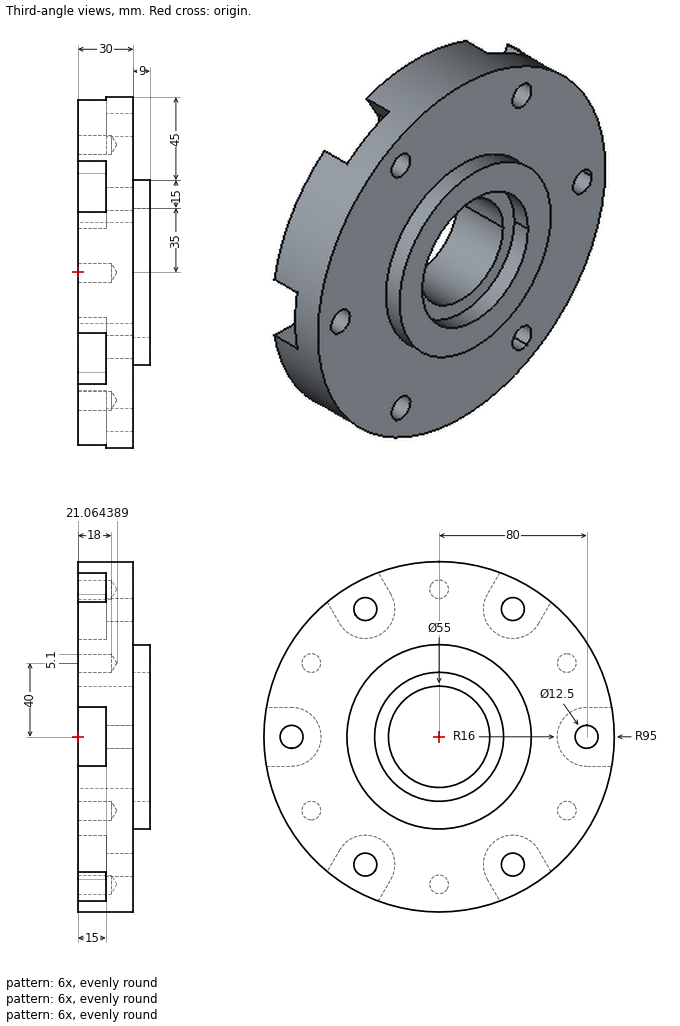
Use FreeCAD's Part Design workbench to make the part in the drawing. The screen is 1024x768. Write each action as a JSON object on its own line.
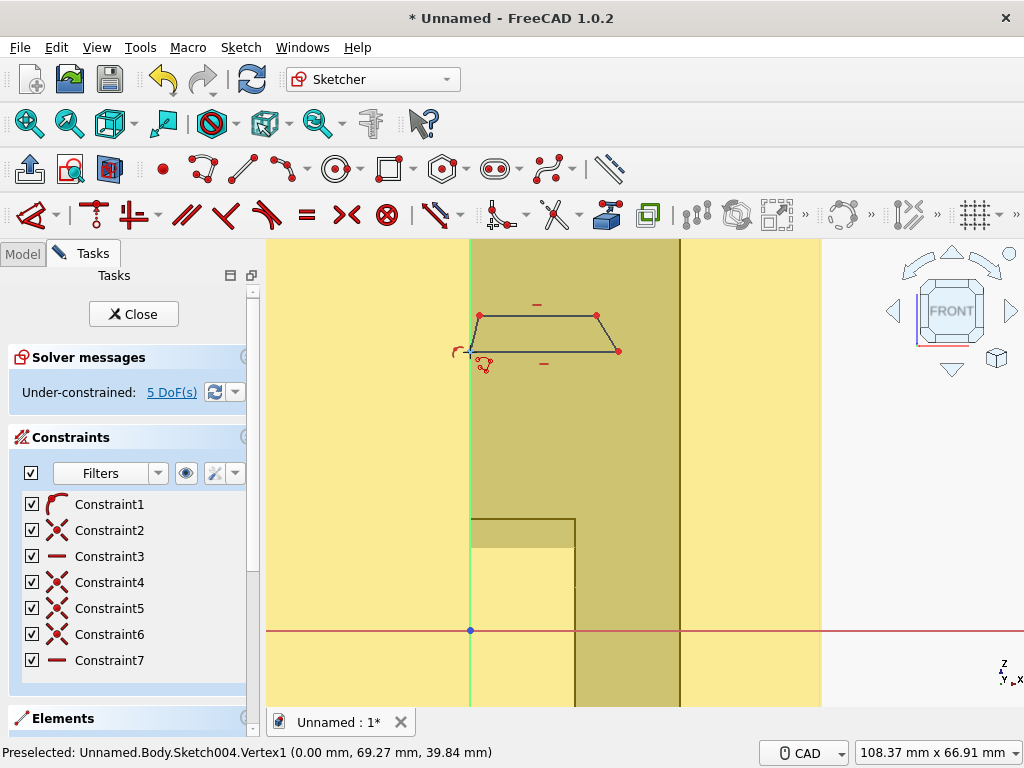
{"action": "left_click", "coordinate": [244, 170]}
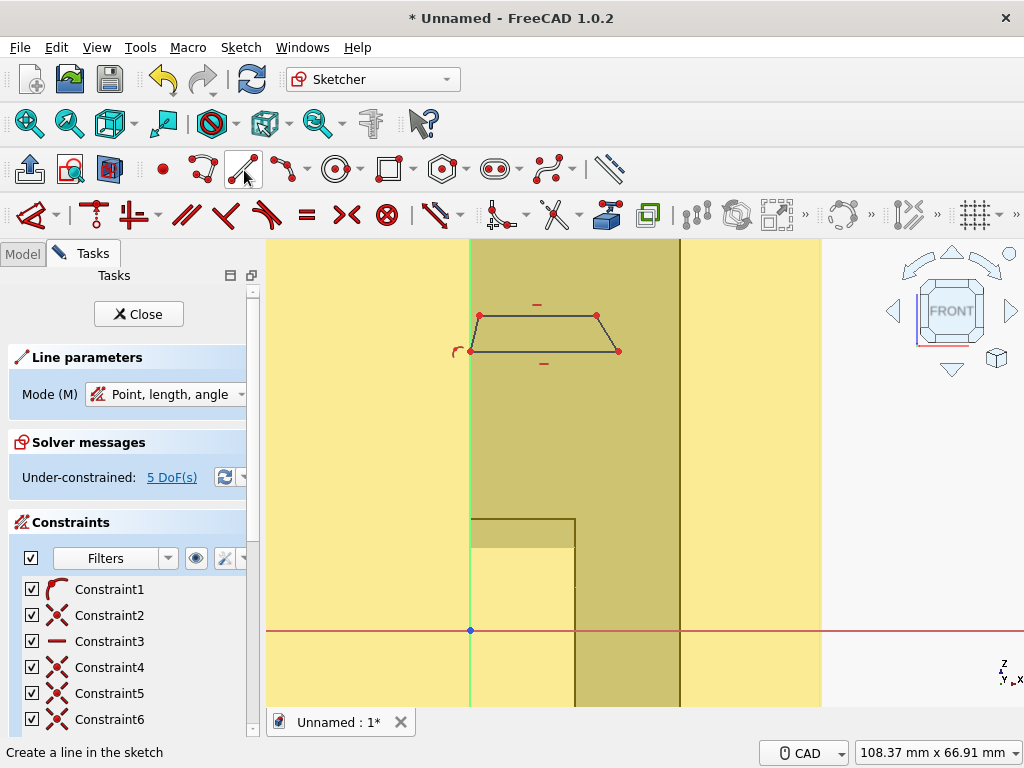
{"action": "left_click", "coordinate": [632, 351]}
{"action": "left_click", "coordinate": [677, 351]}
{"action": "key", "text": "Escape"}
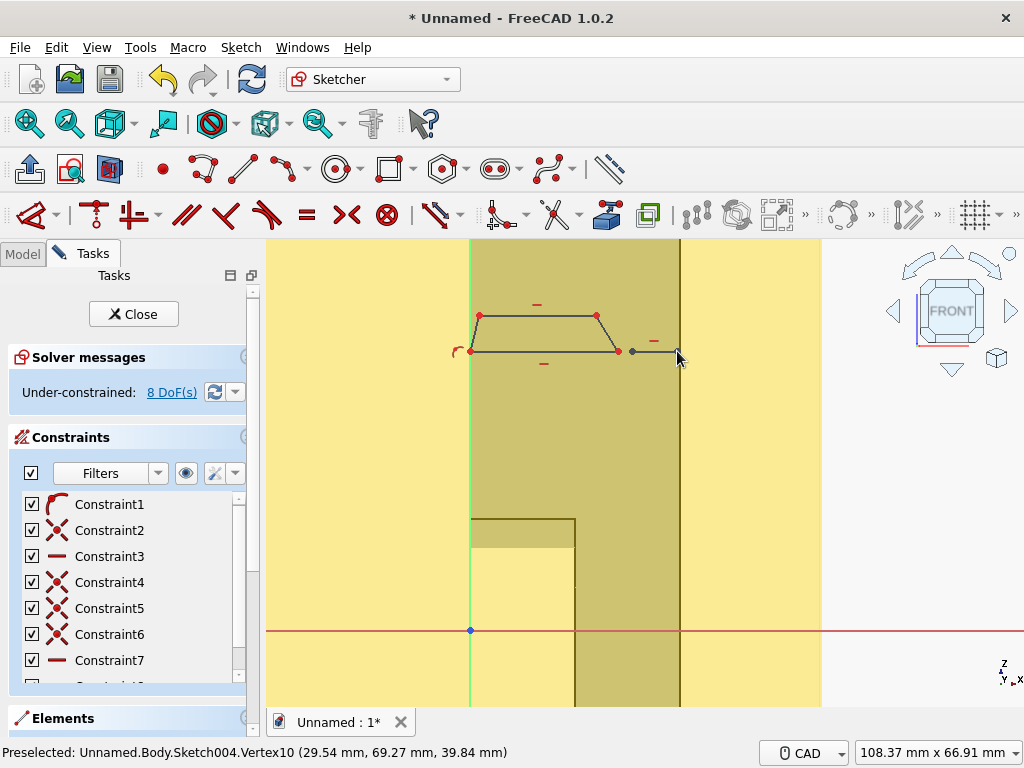
{"action": "left_click", "coordinate": [645, 352]}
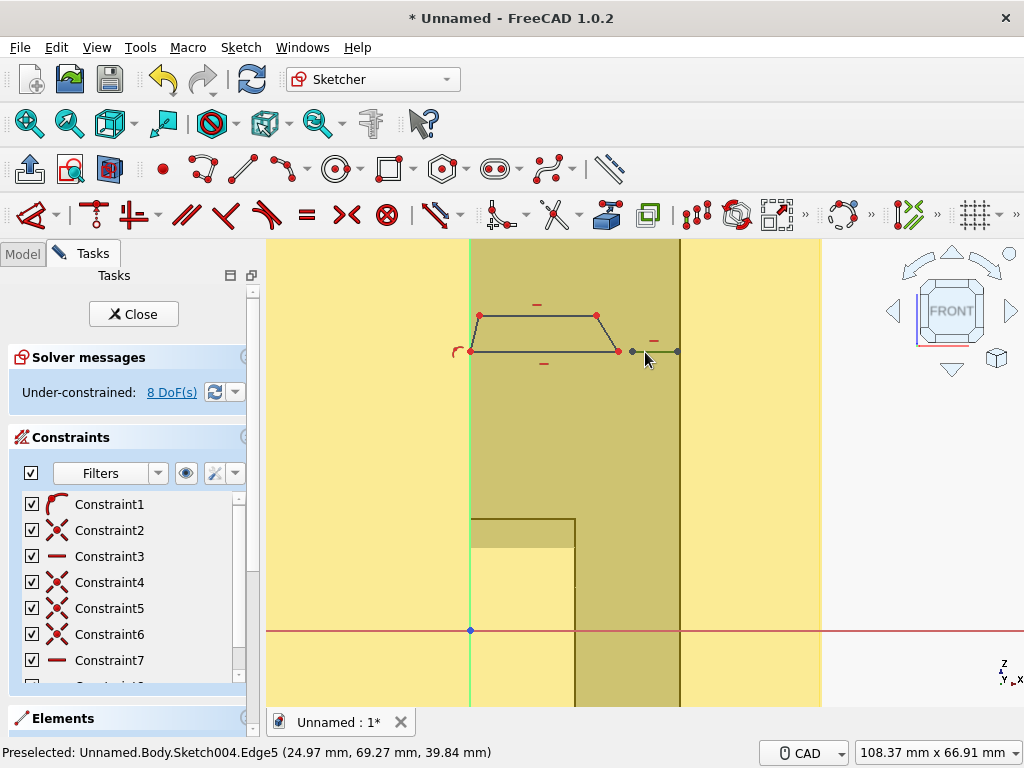
{"action": "left_click", "coordinate": [610, 170]}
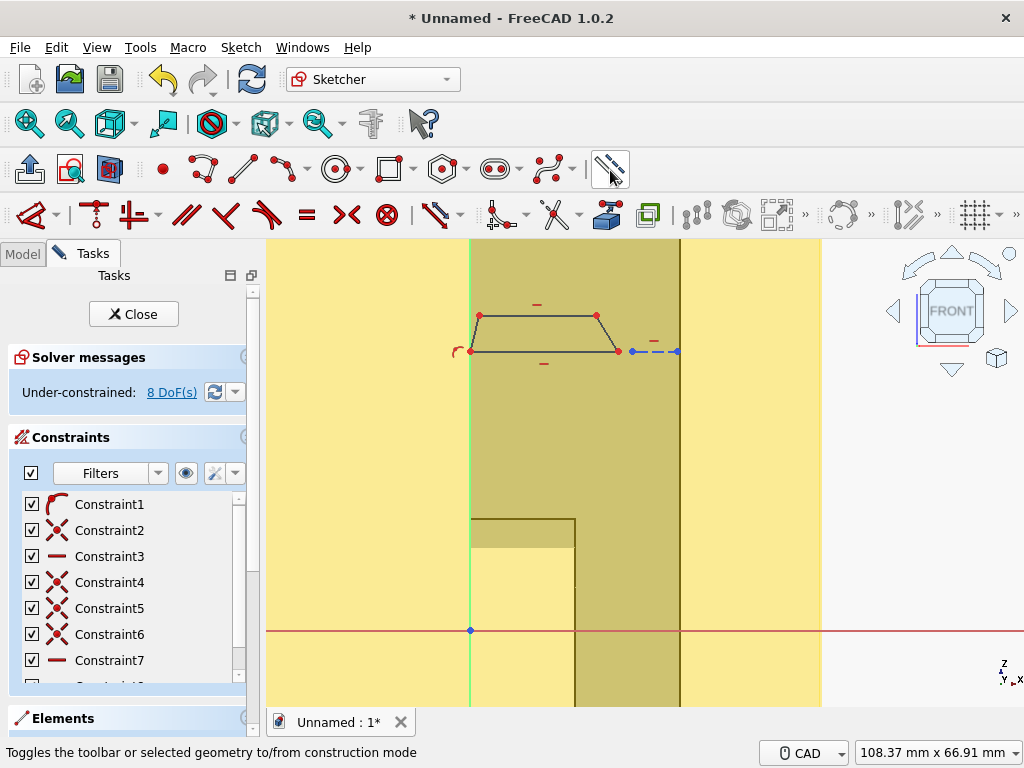
{"action": "scroll", "coordinate": [473, 341], "scroll_direction": "up", "scroll_amount": 2}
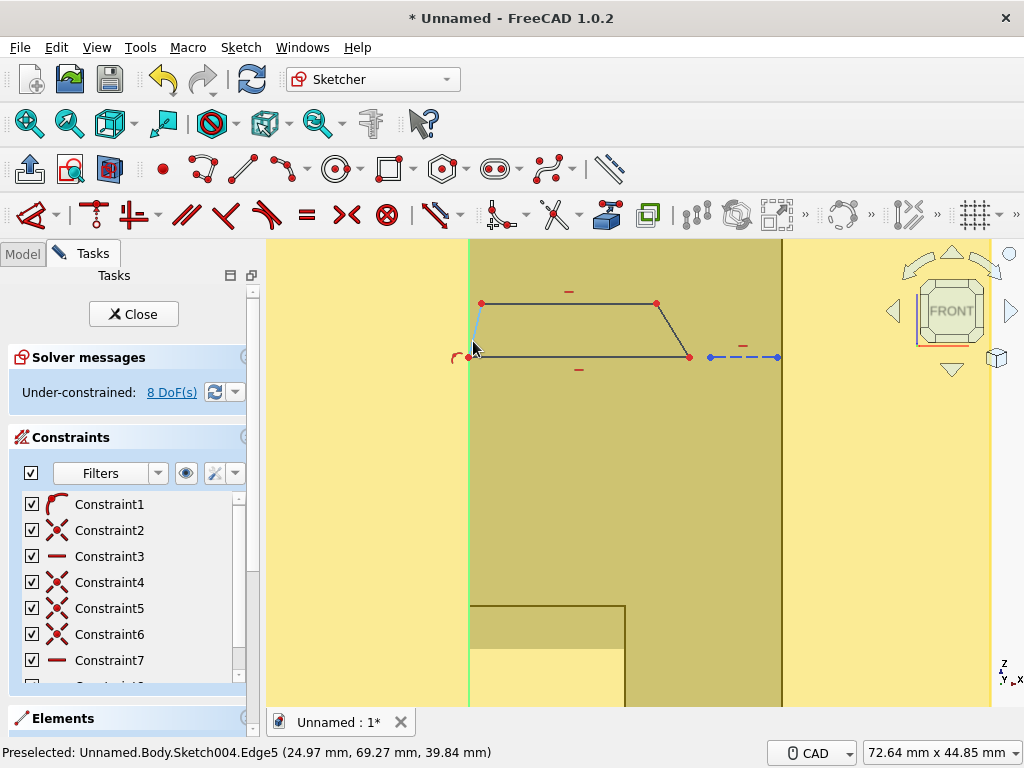
{"action": "left_click", "coordinate": [473, 341]}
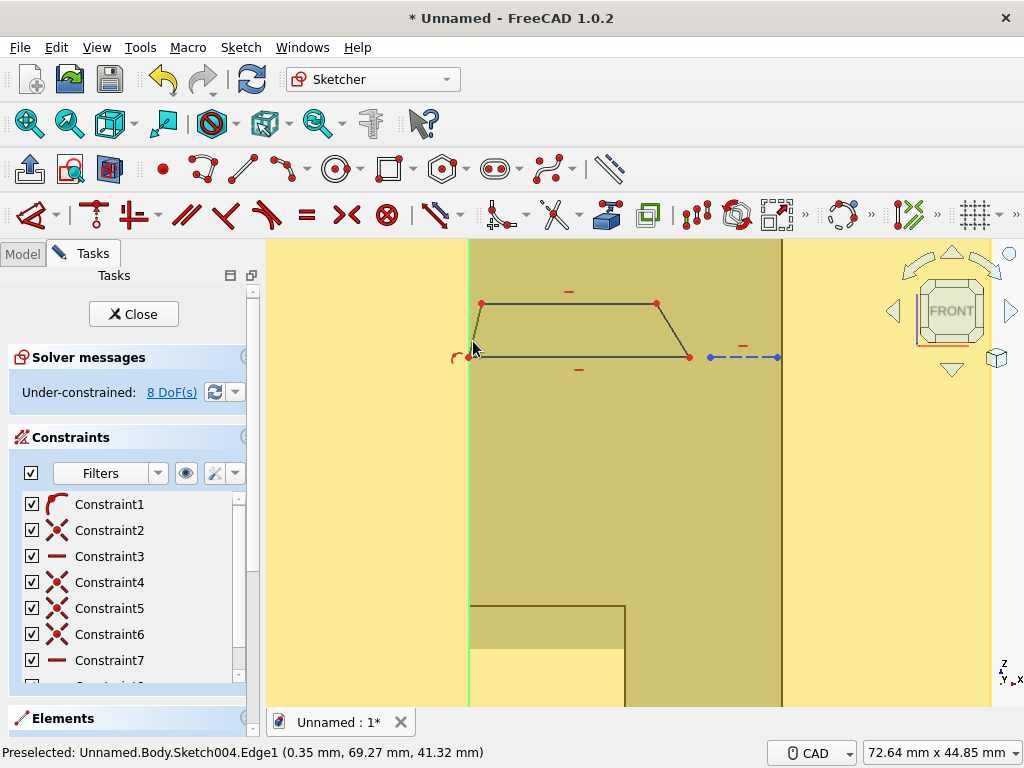
{"action": "left_click", "coordinate": [160, 216]}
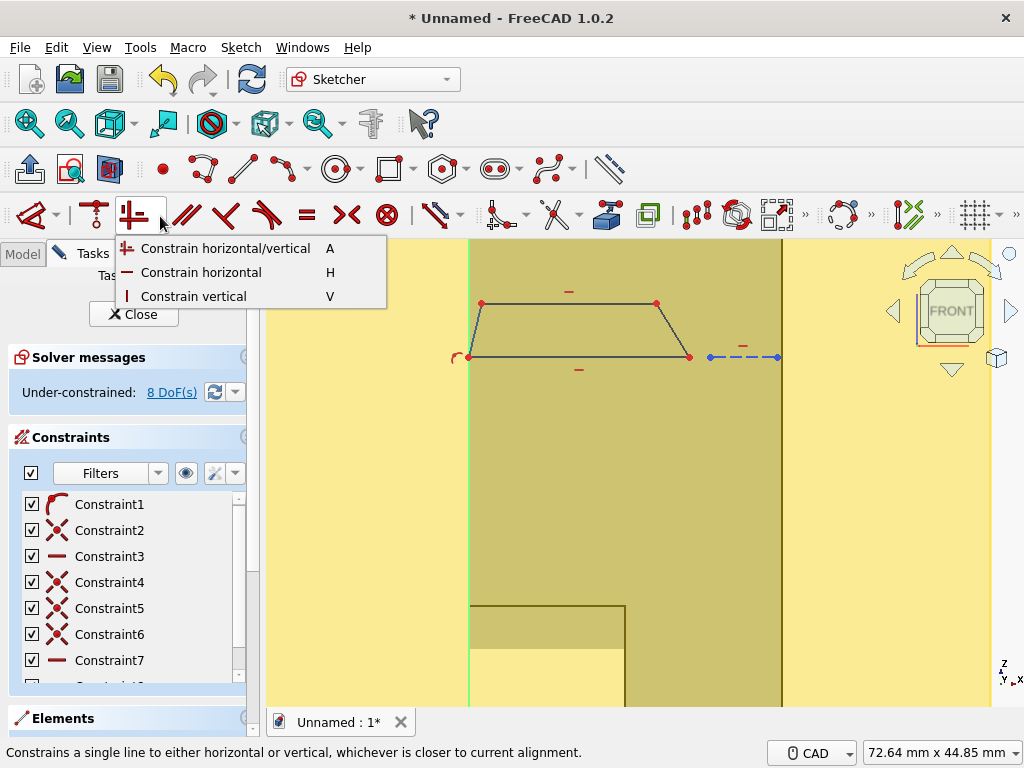
{"action": "left_click", "coordinate": [251, 296]}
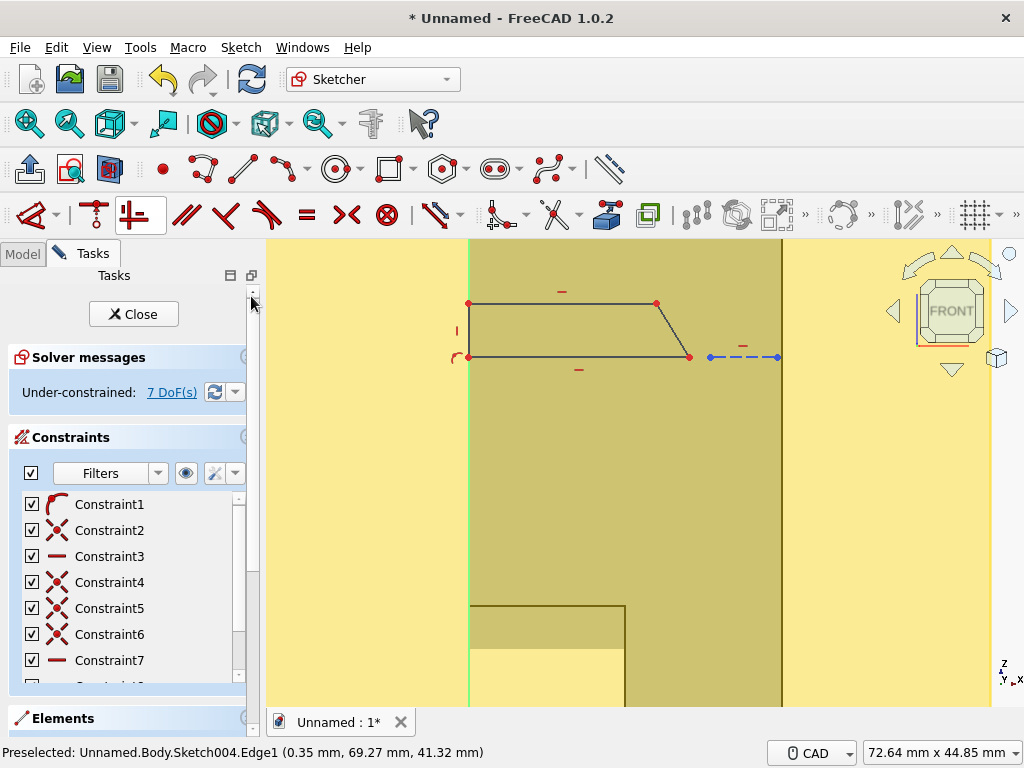
{"action": "key", "text": "d"}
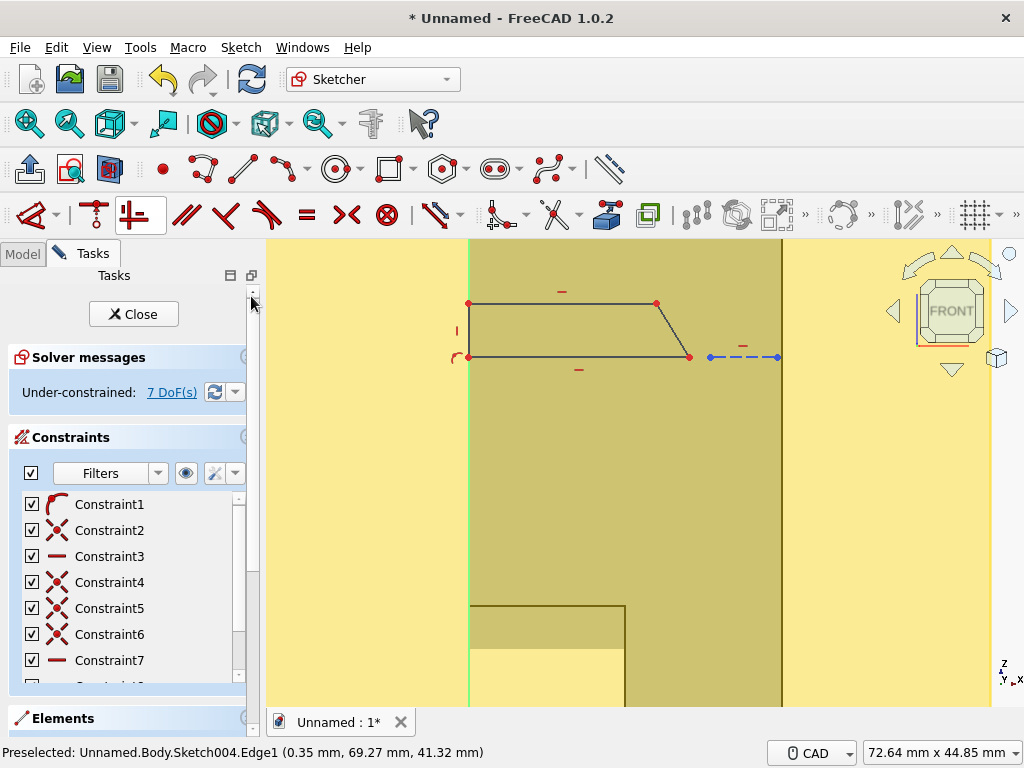
{"action": "left_click", "coordinate": [525, 304]}
{"action": "left_click", "coordinate": [563, 270]}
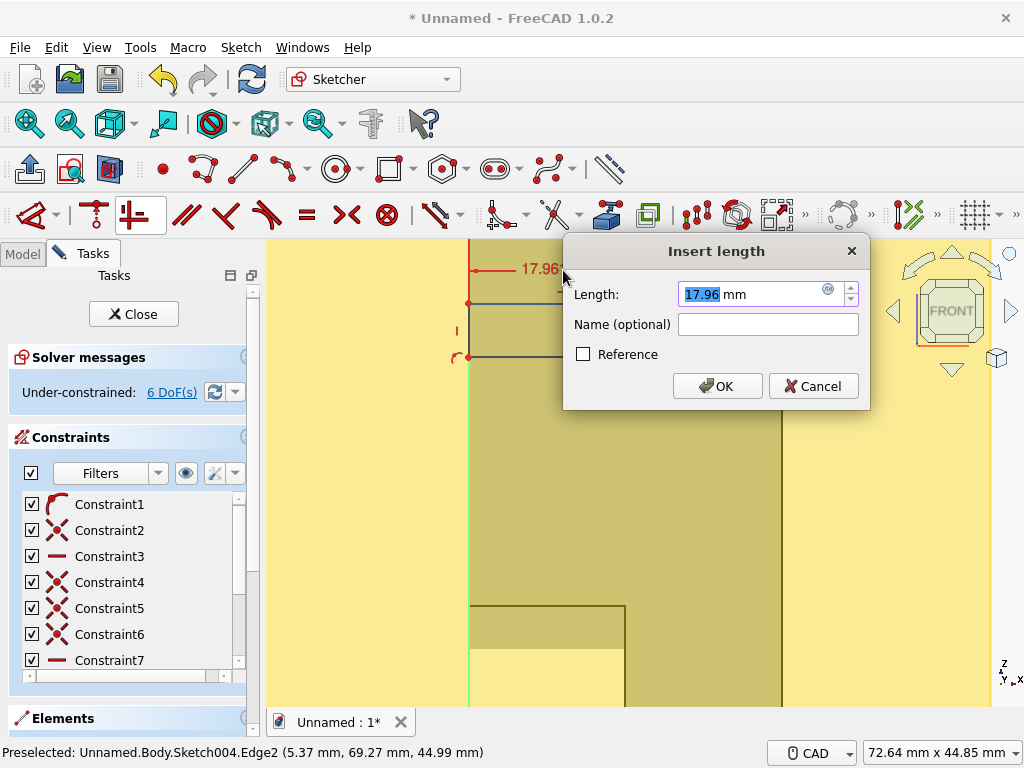
{"action": "type", "text": "18"}
{"action": "key", "text": "Return"}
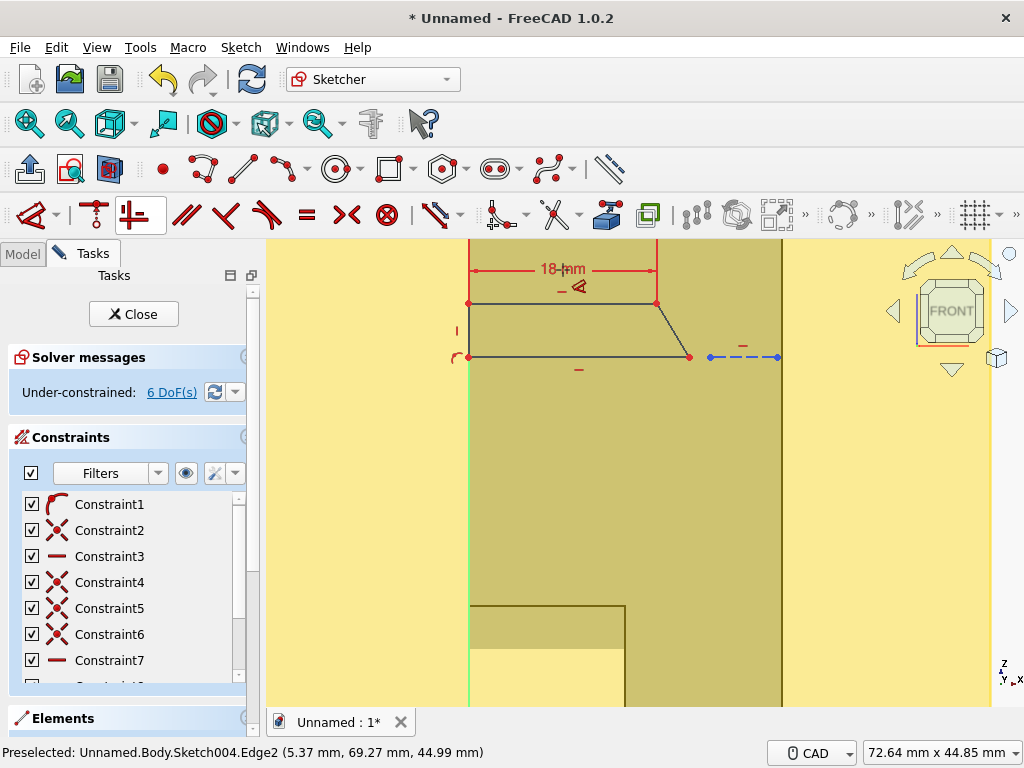
{"action": "left_click", "coordinate": [469, 341]}
{"action": "left_click", "coordinate": [435, 330]}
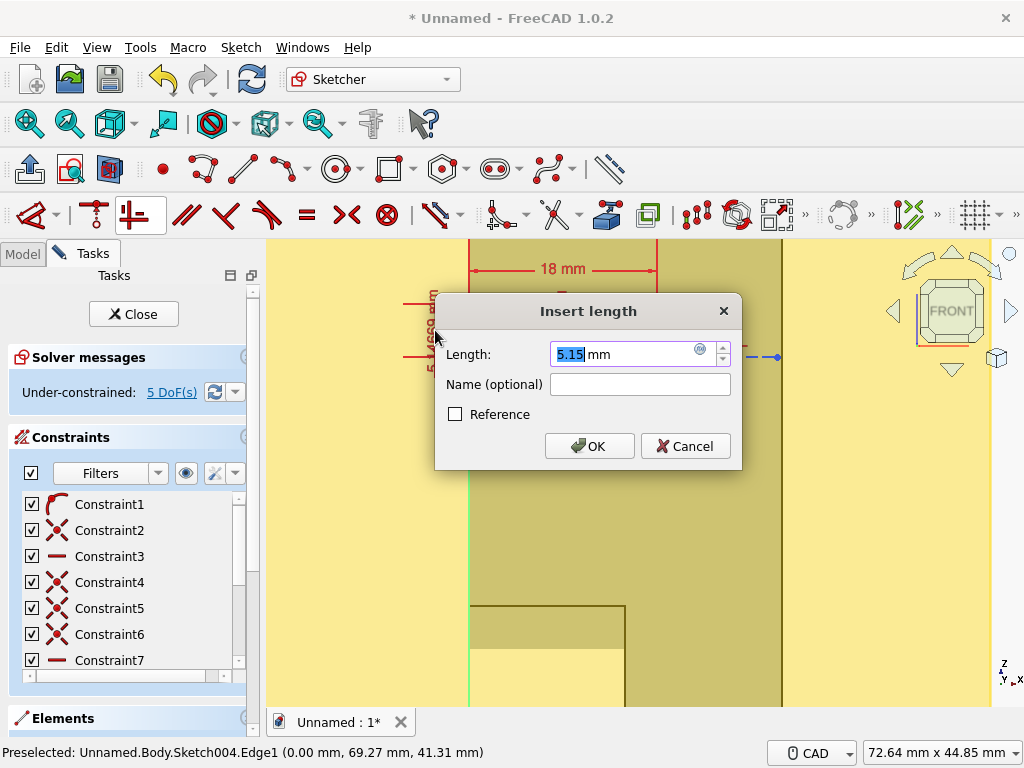
{"action": "type", "text": "5.1"}
{"action": "key", "text": "Return"}